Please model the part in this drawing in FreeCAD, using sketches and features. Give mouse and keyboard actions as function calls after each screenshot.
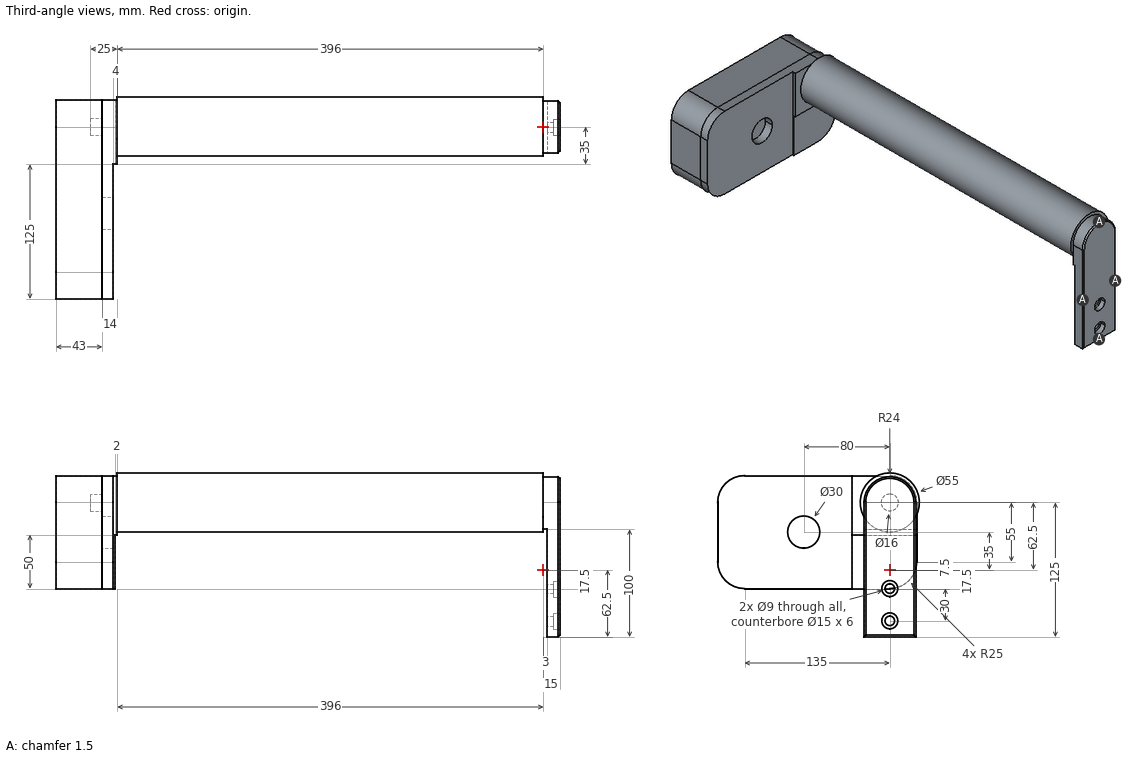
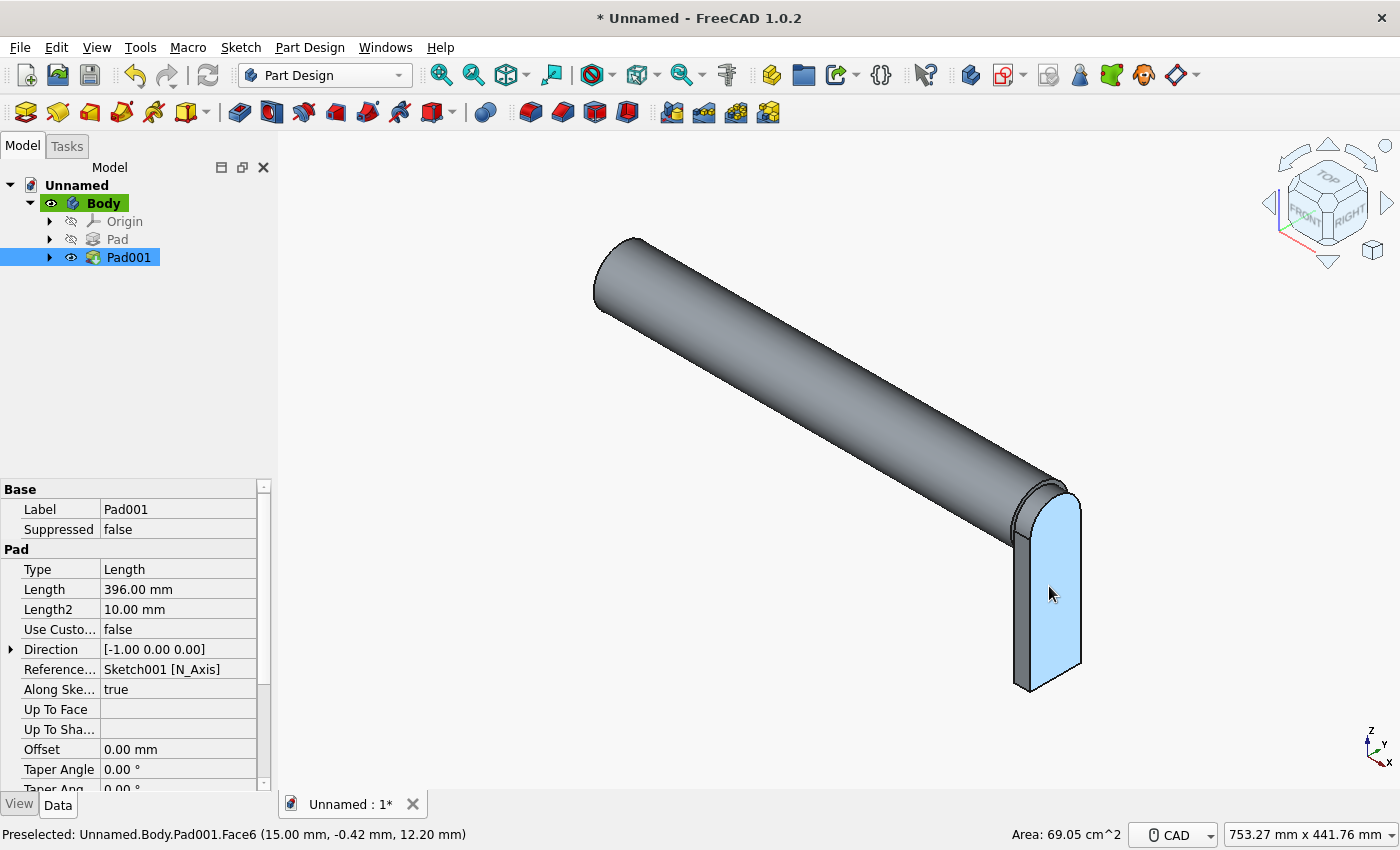
click(1004, 76)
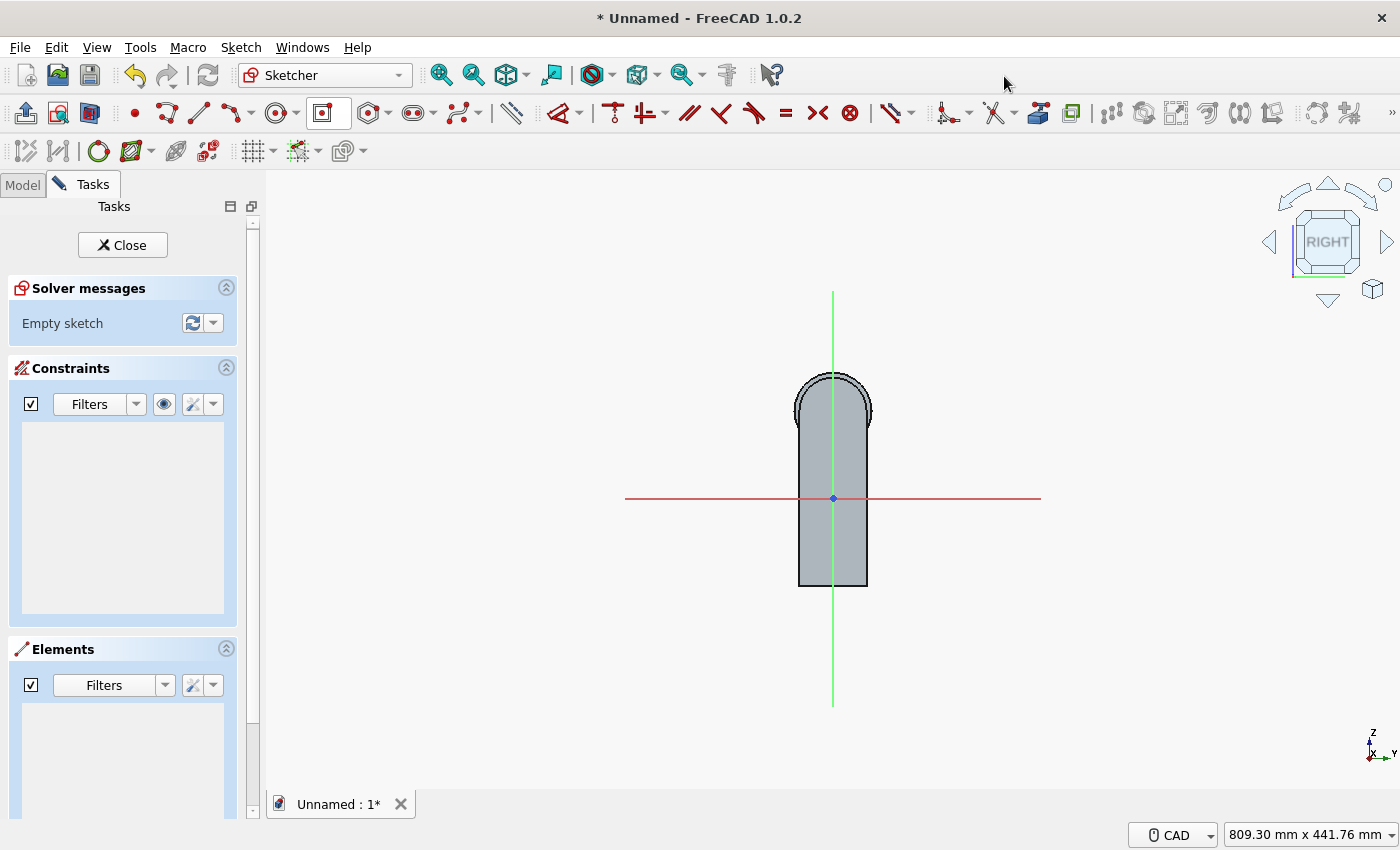
scroll(850, 549, up, 8)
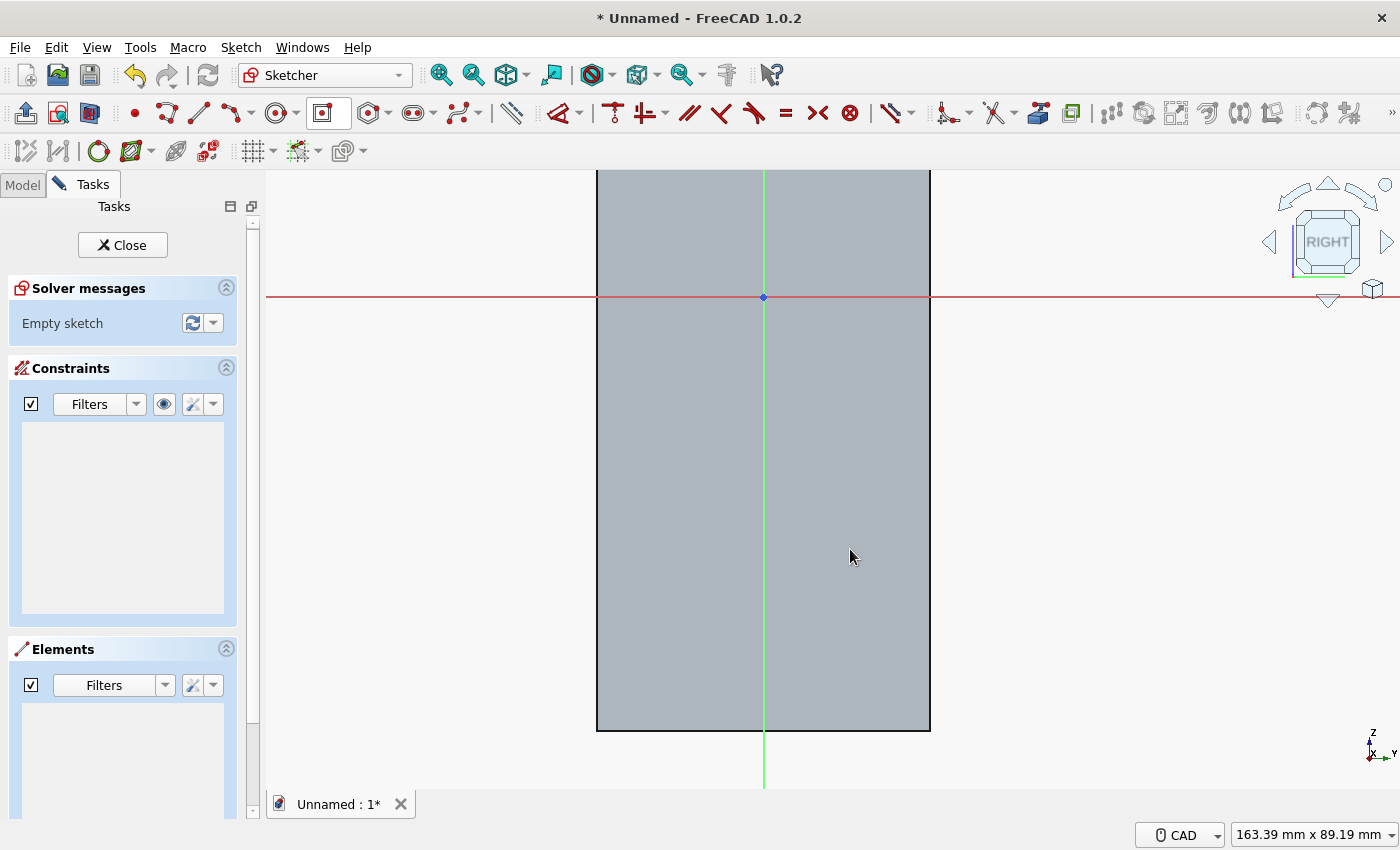
key(g)
key(c)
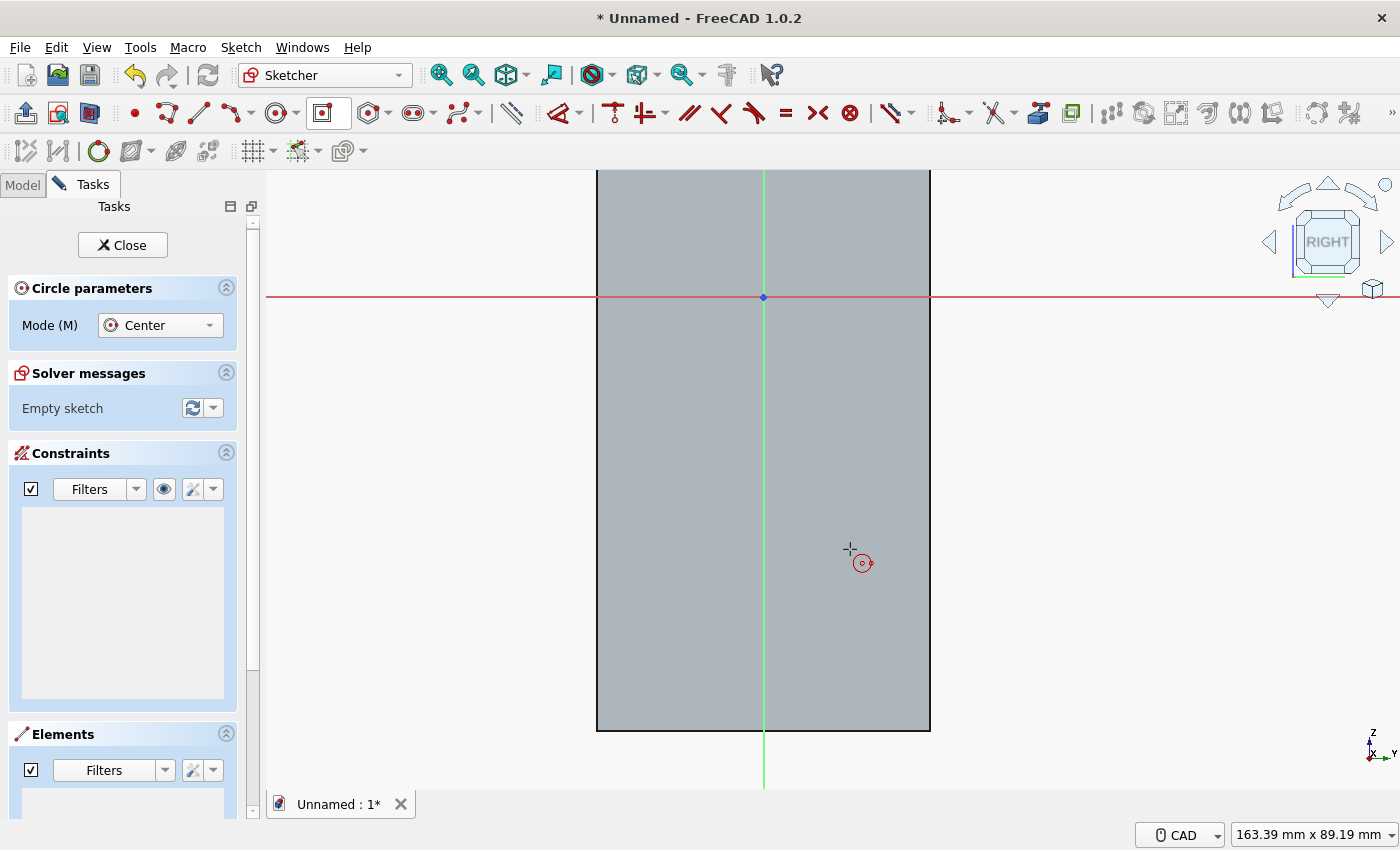
click(764, 419)
move(786, 397)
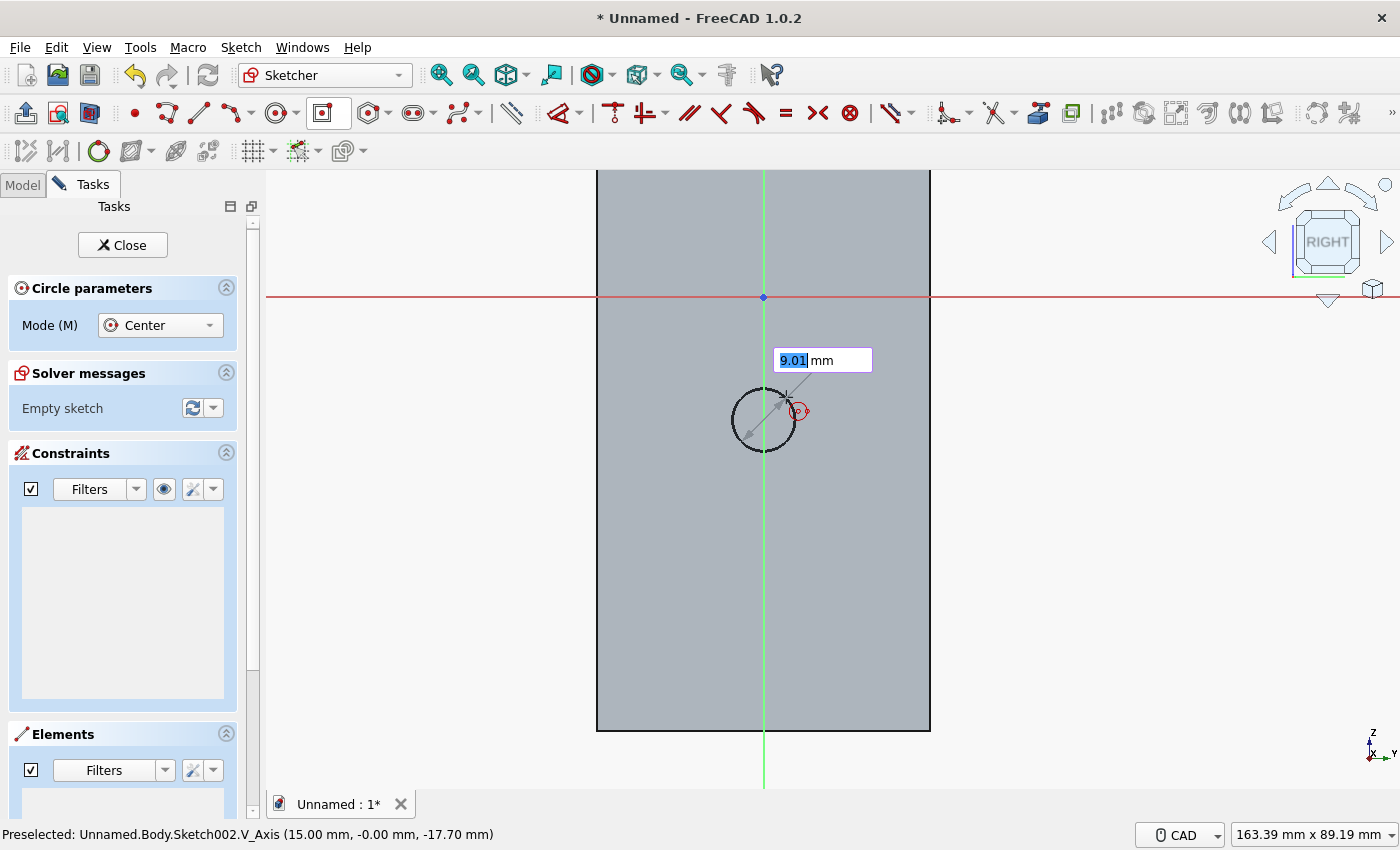
text(9)
key(Return)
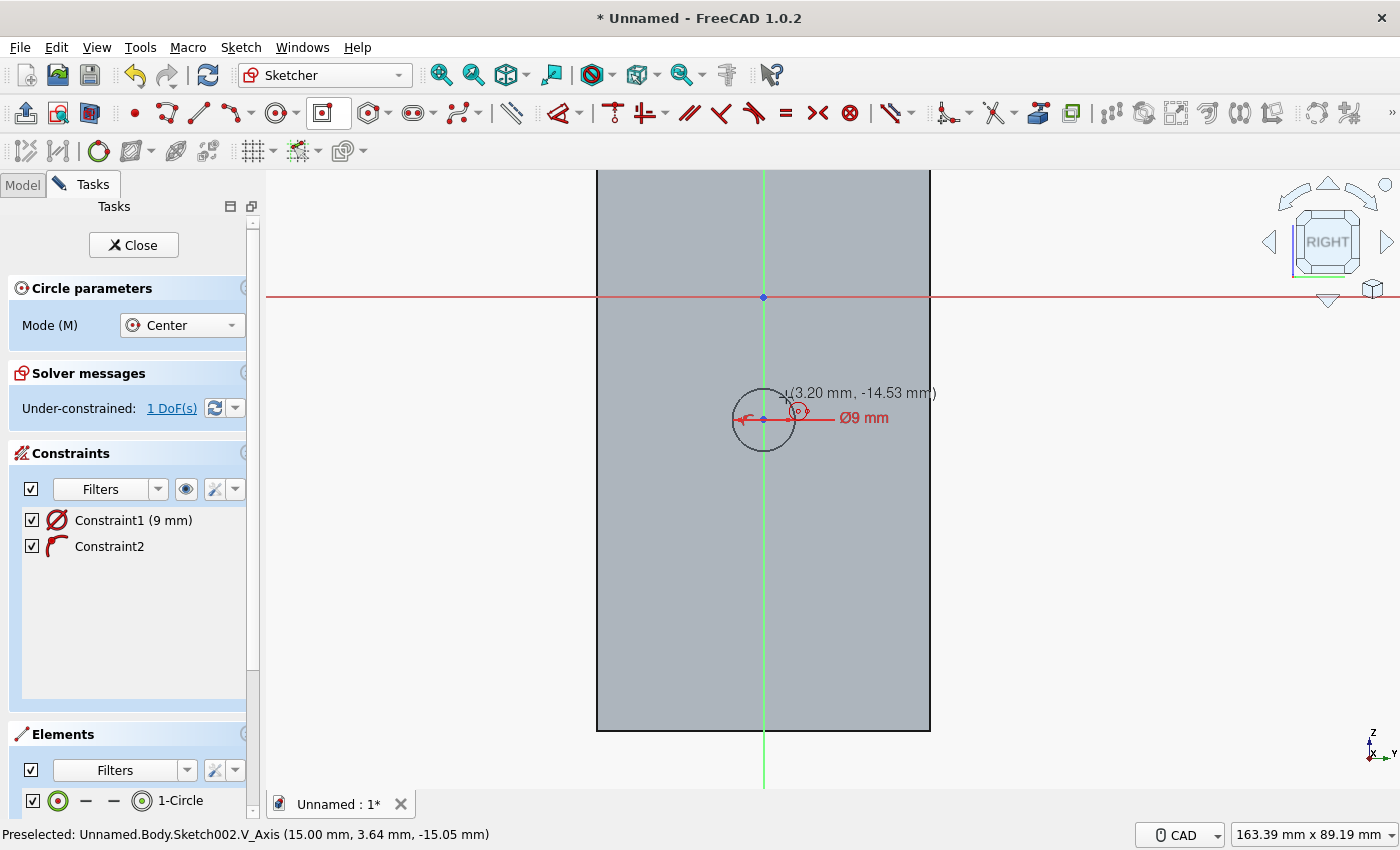
click(764, 627)
move(786, 605)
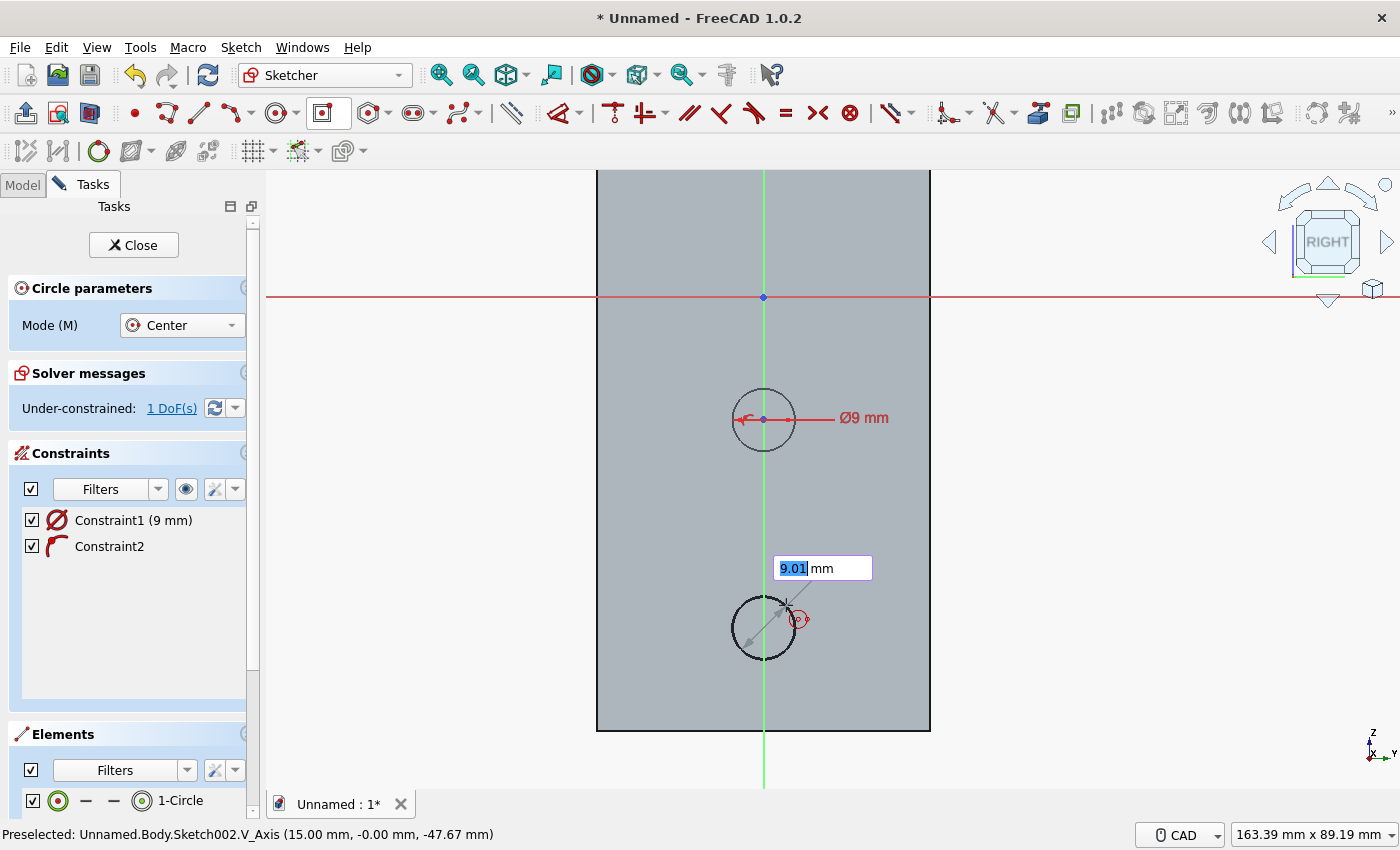
text(9)
key(Return)
key(Escape)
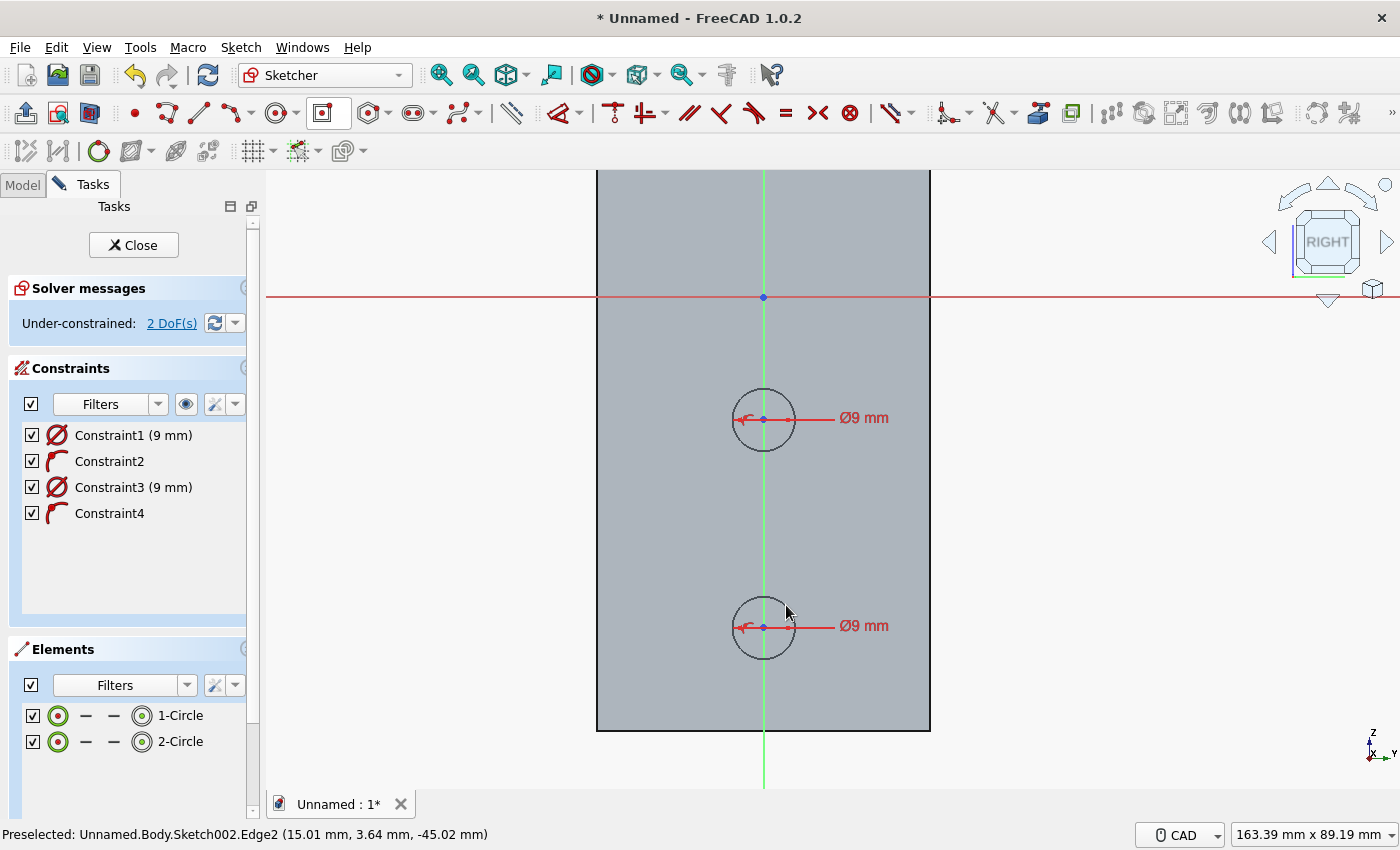
key(d)